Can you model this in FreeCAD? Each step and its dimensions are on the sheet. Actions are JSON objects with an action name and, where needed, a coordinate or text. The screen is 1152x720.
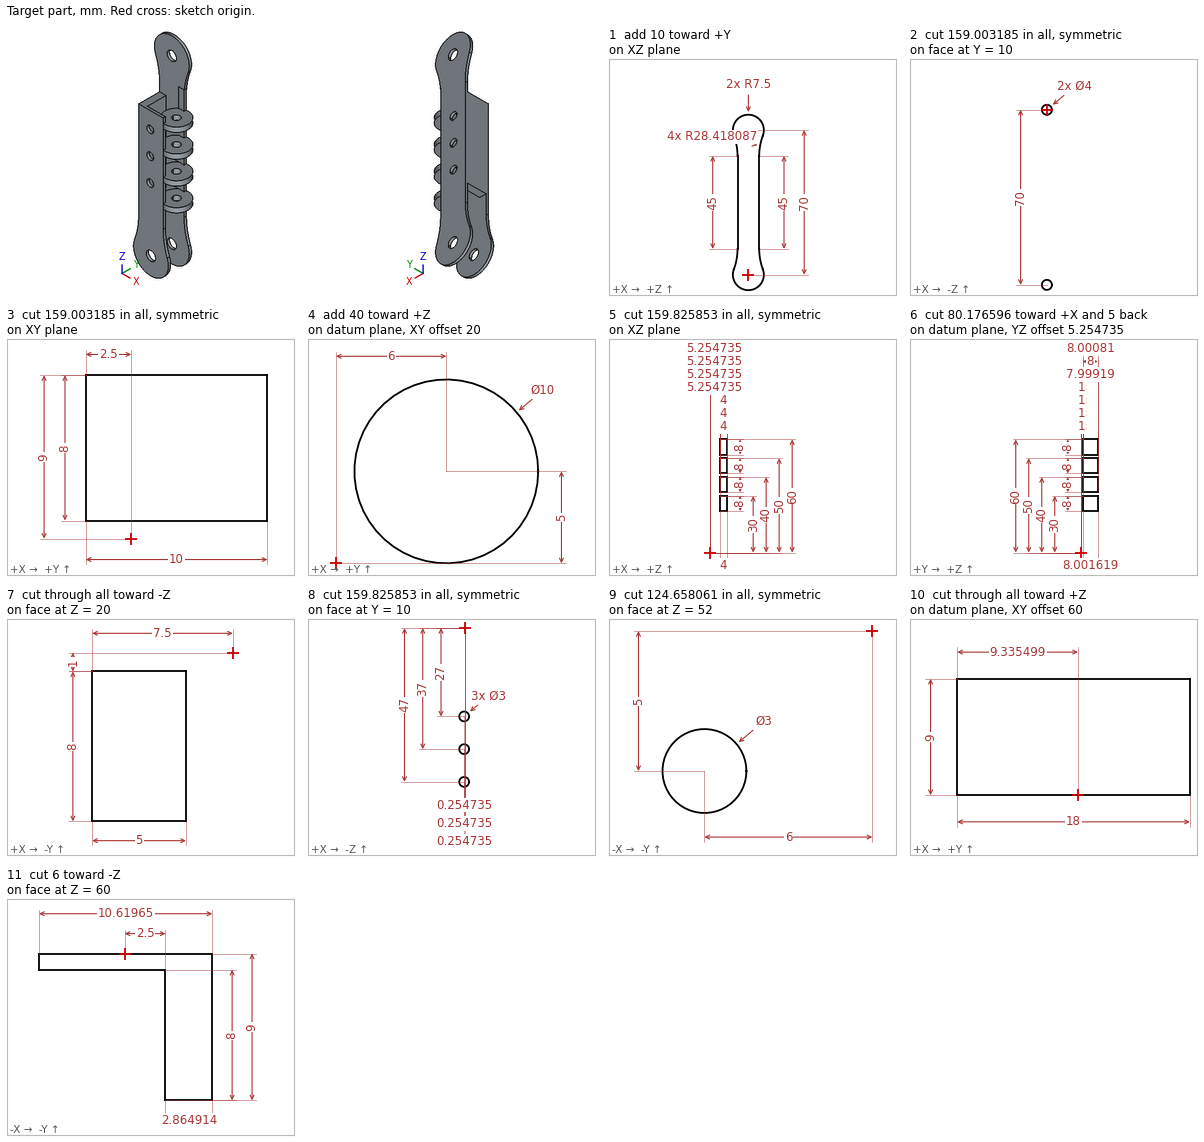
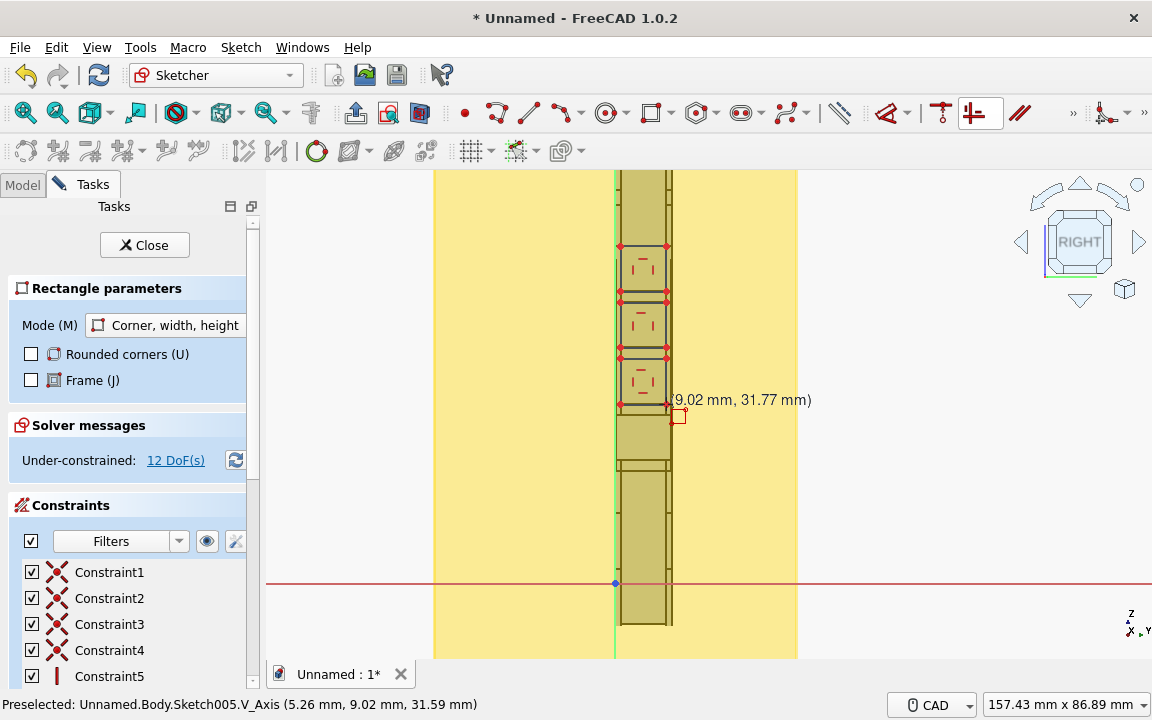
{"action": "scroll", "coordinate": [621, 415], "scroll_direction": "up", "scroll_amount": 6}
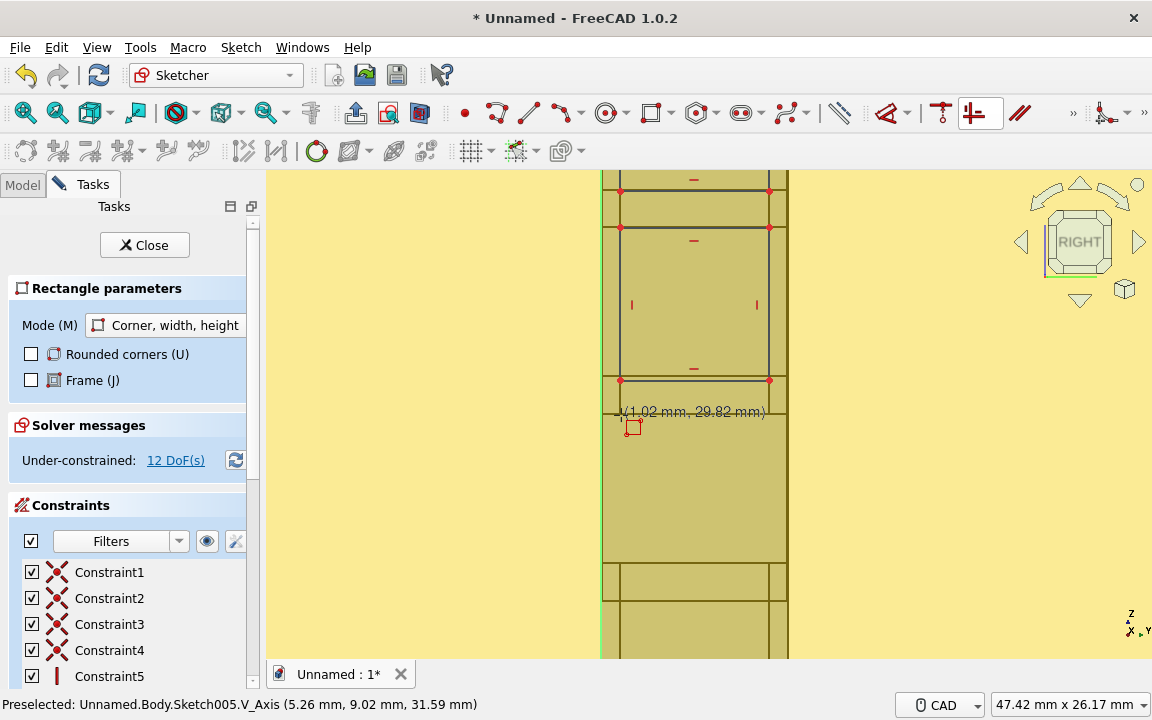
{"action": "left_click", "coordinate": [620, 414]}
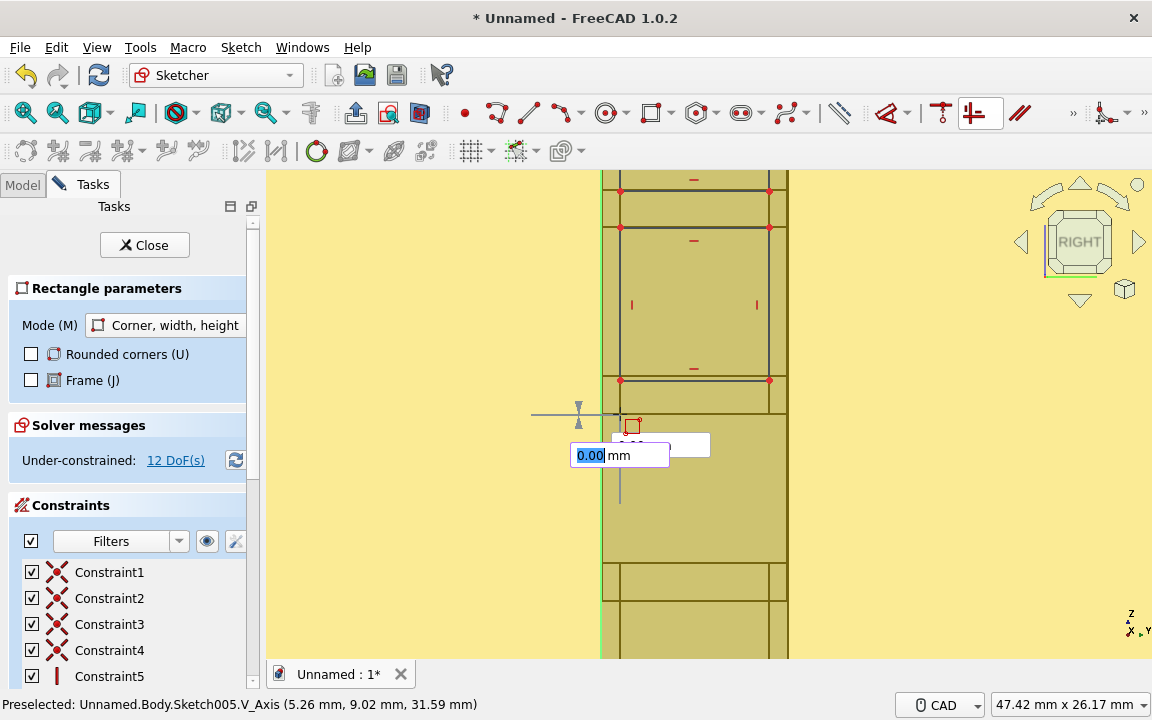
{"action": "scroll", "coordinate": [621, 415], "scroll_direction": "down", "scroll_amount": 6}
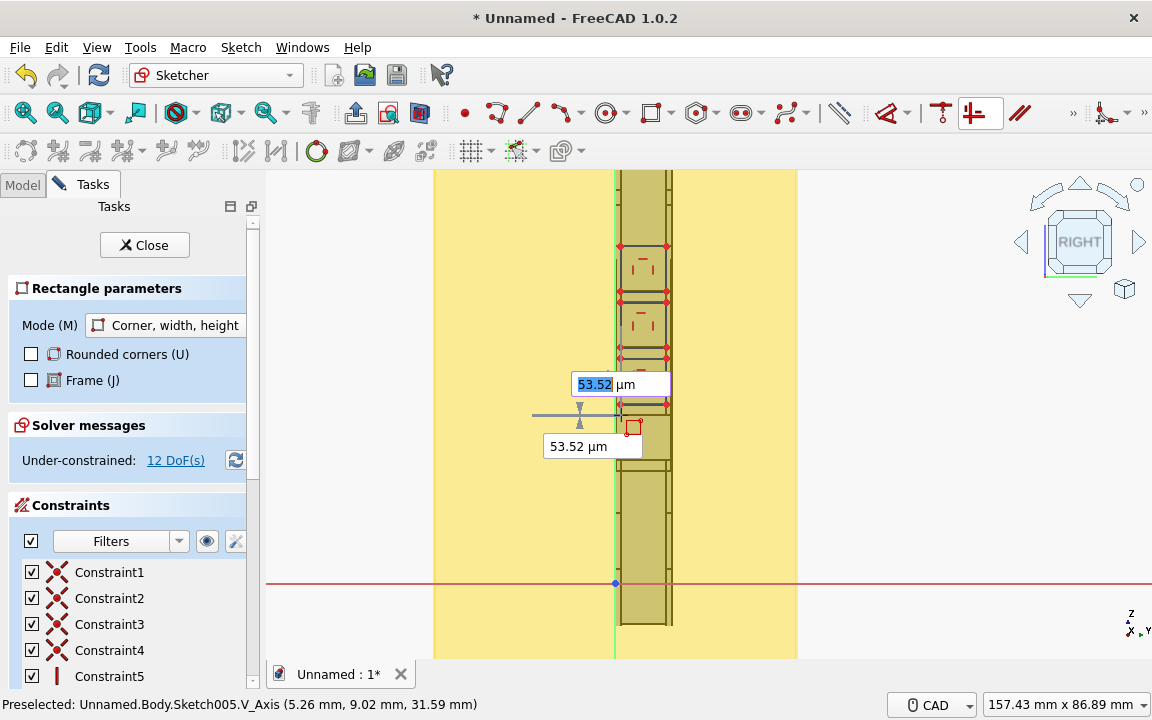
{"action": "left_click", "coordinate": [666, 460]}
{"action": "key", "text": "Escape"}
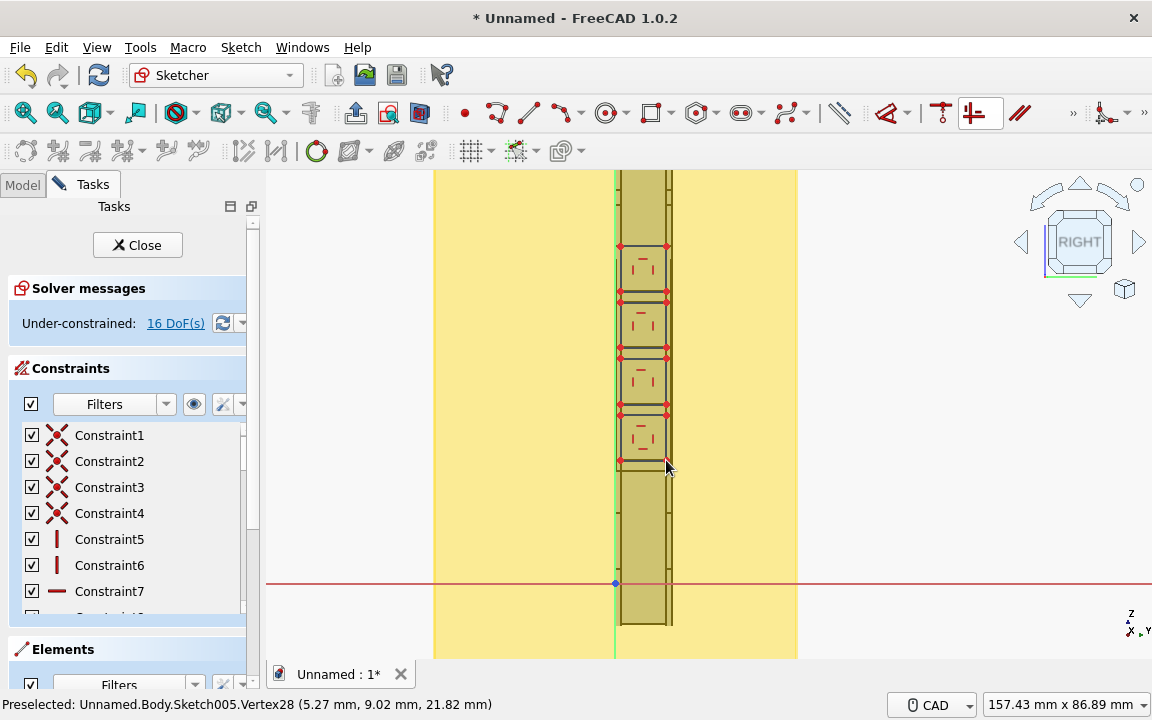
{"action": "scroll", "coordinate": [621, 260], "scroll_direction": "up", "scroll_amount": 5}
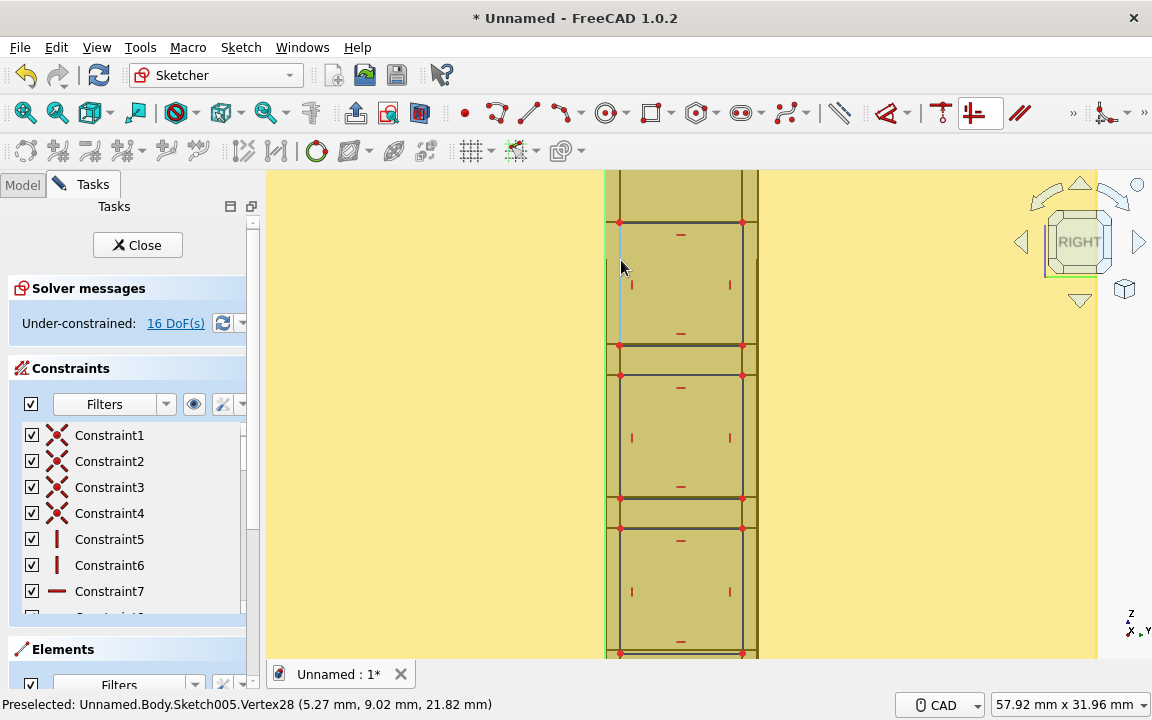
{"action": "left_click", "coordinate": [620, 260]}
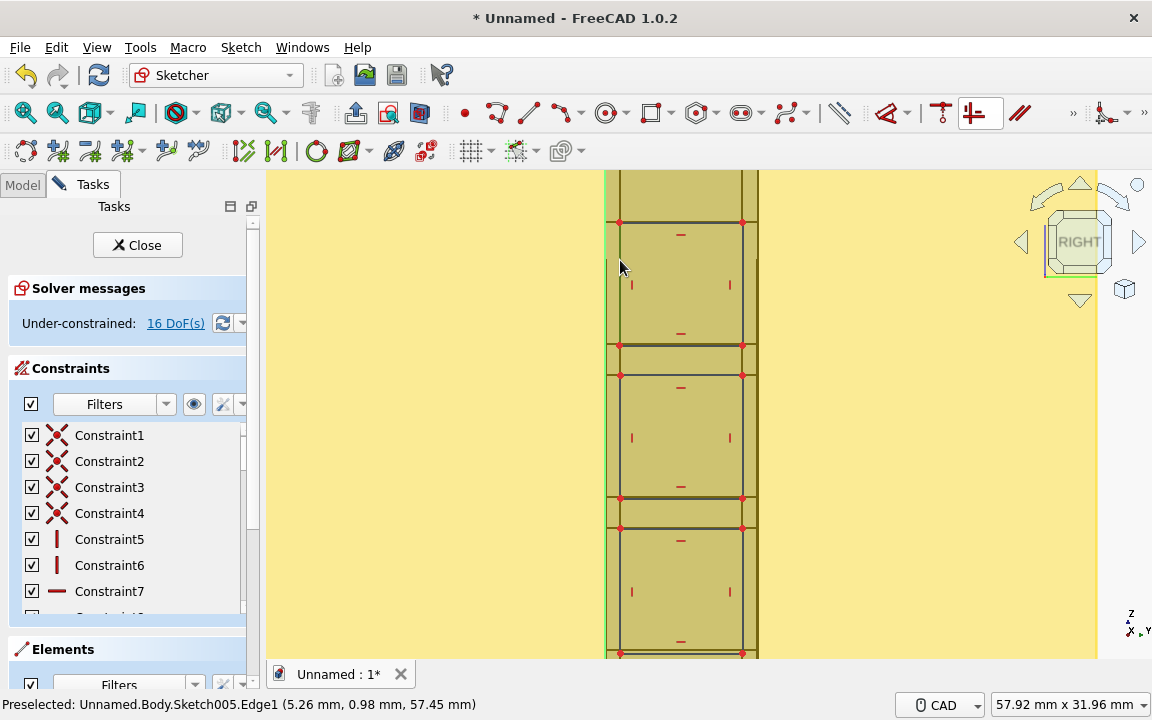
{"action": "key", "text": "i"}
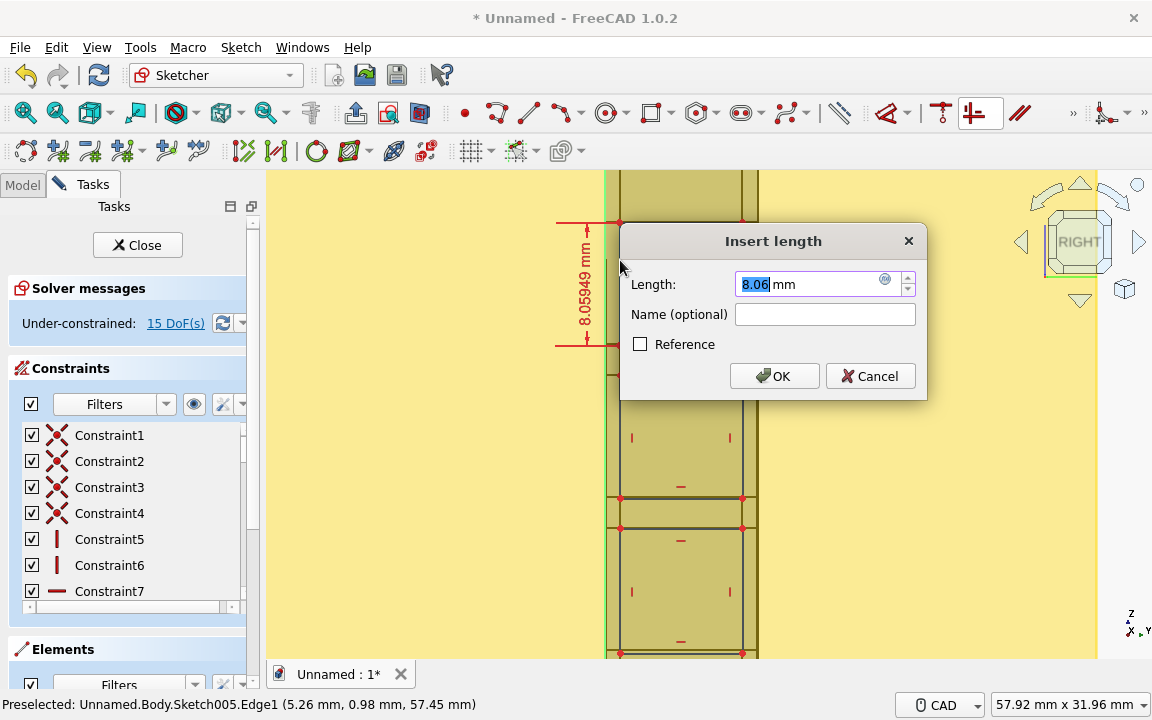
{"action": "type", "text": "8"}
{"action": "key", "text": "Return"}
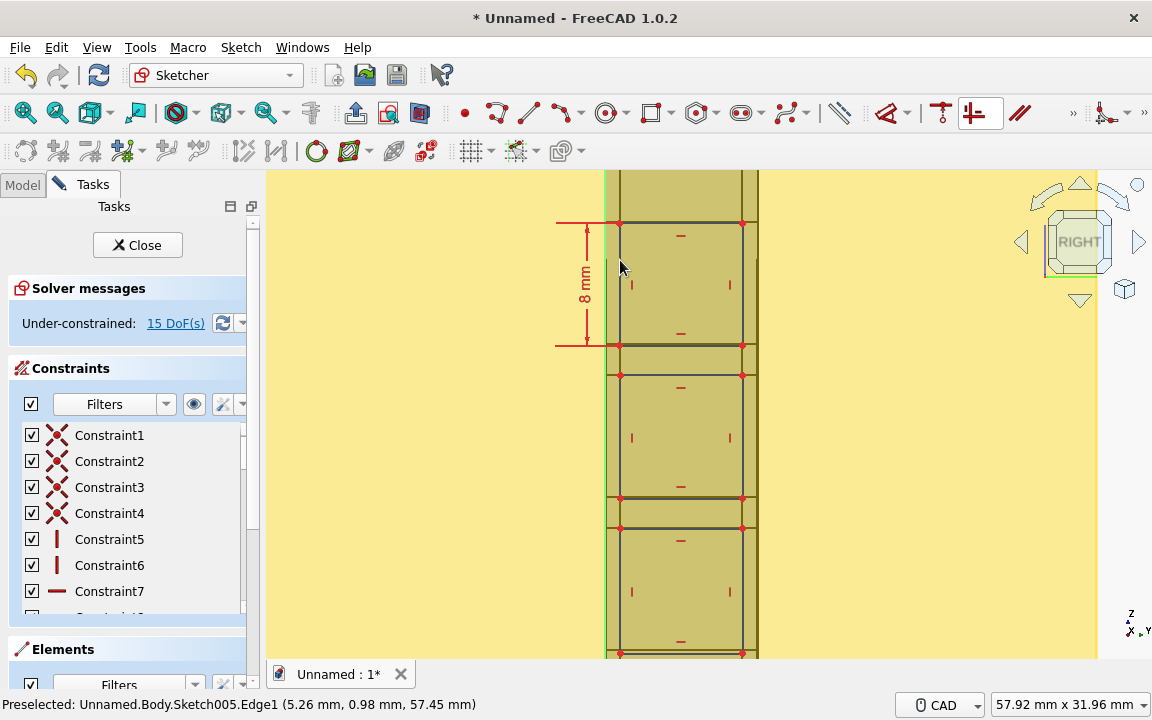
{"action": "left_click", "coordinate": [620, 412]}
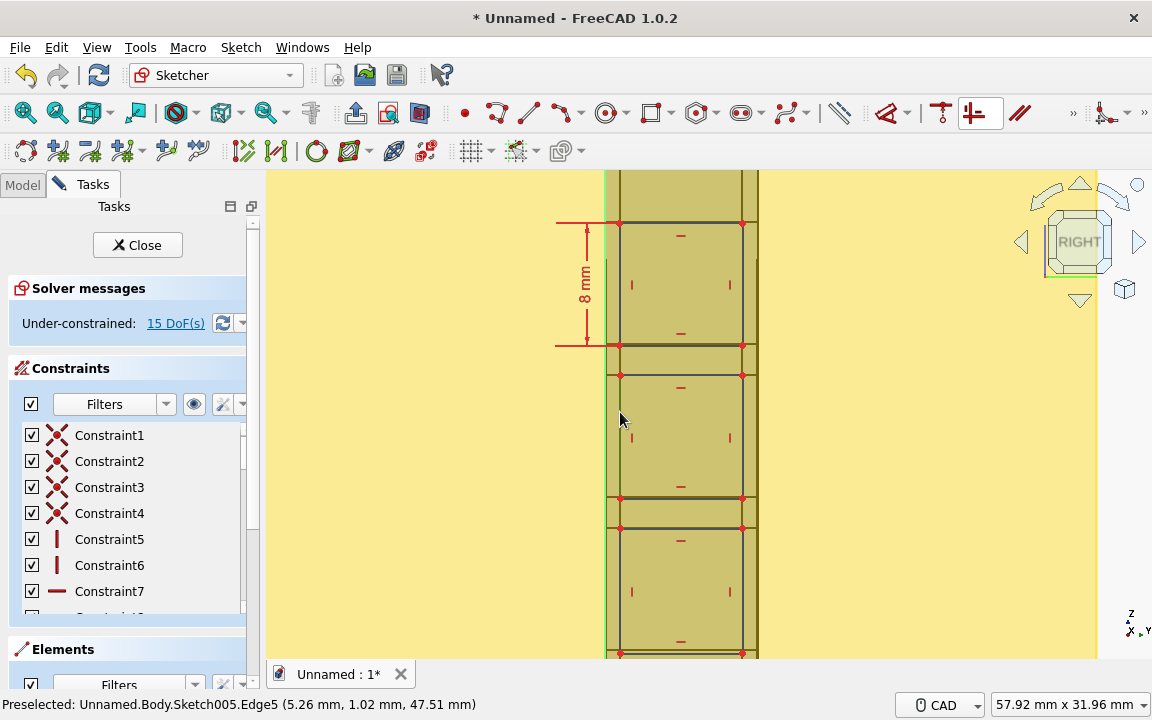
{"action": "key", "text": "i"}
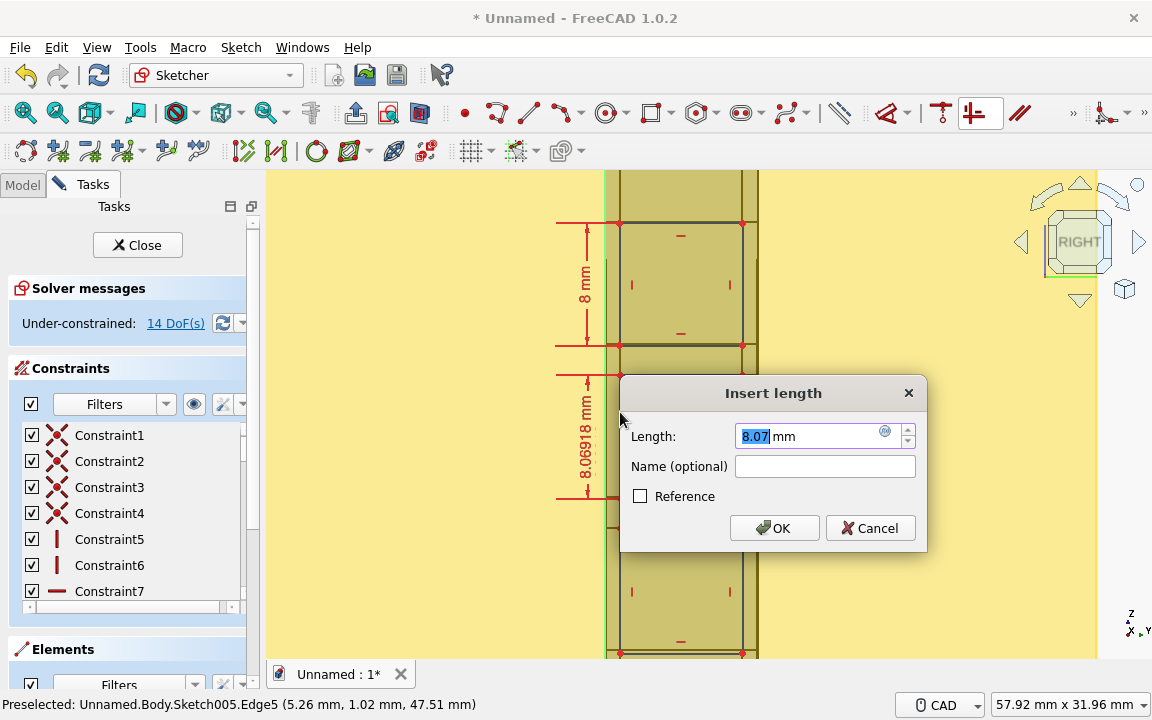
{"action": "type", "text": "8"}
{"action": "key", "text": "Return"}